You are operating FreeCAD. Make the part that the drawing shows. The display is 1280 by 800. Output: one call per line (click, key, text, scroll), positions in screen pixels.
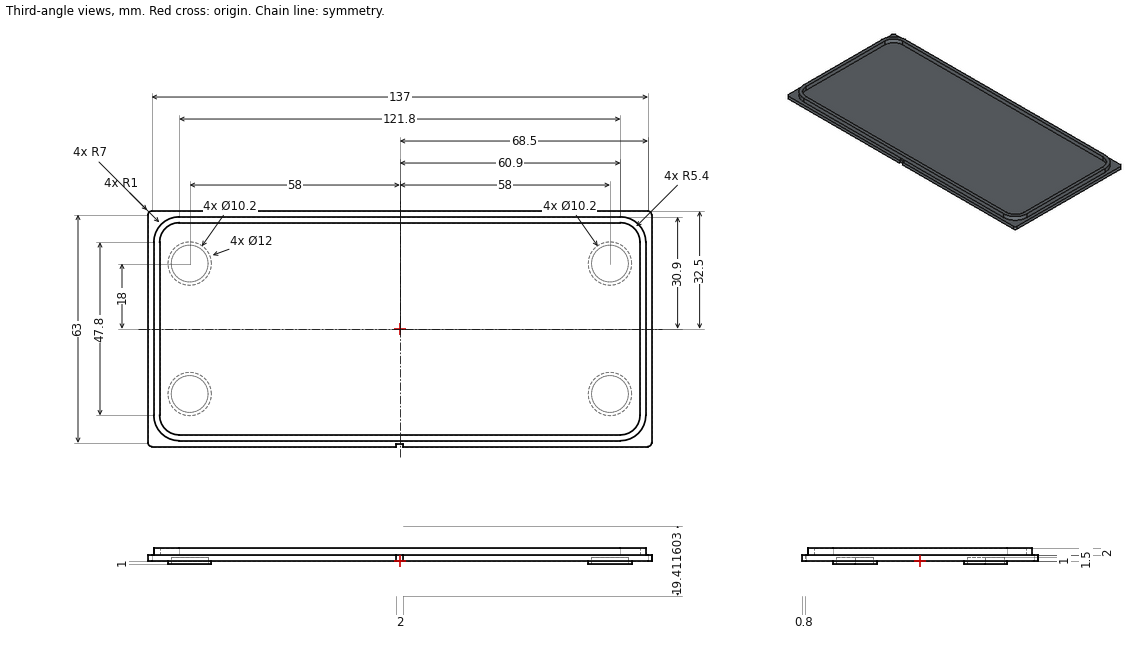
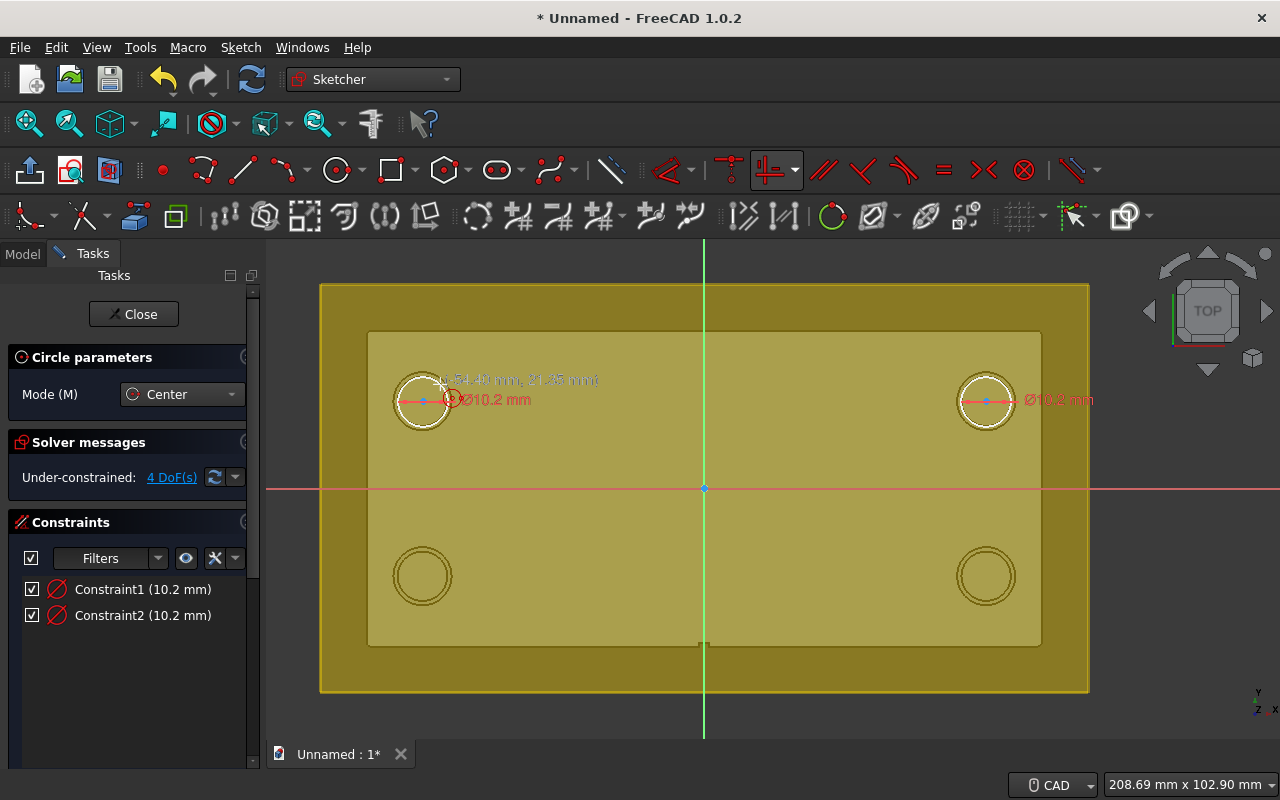
click(423, 576)
move(440, 559)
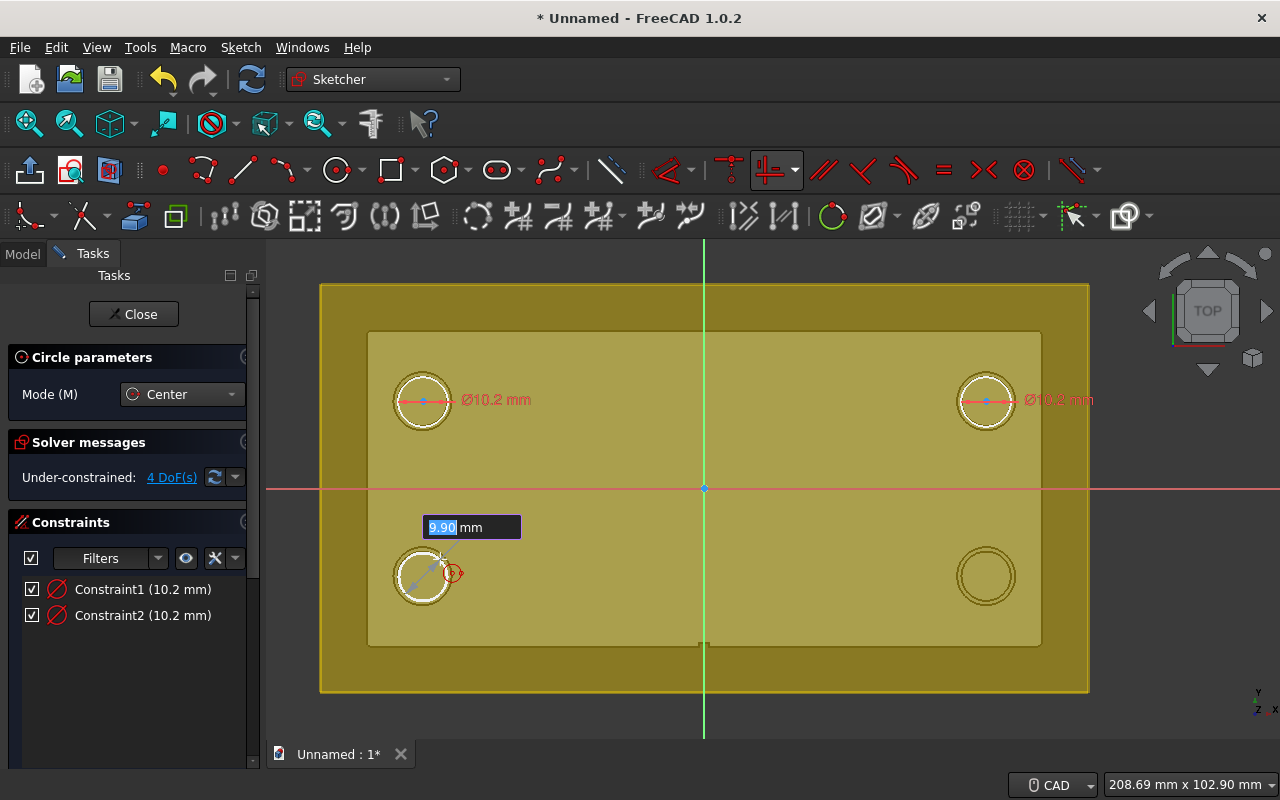
text(10.2)
key(Return)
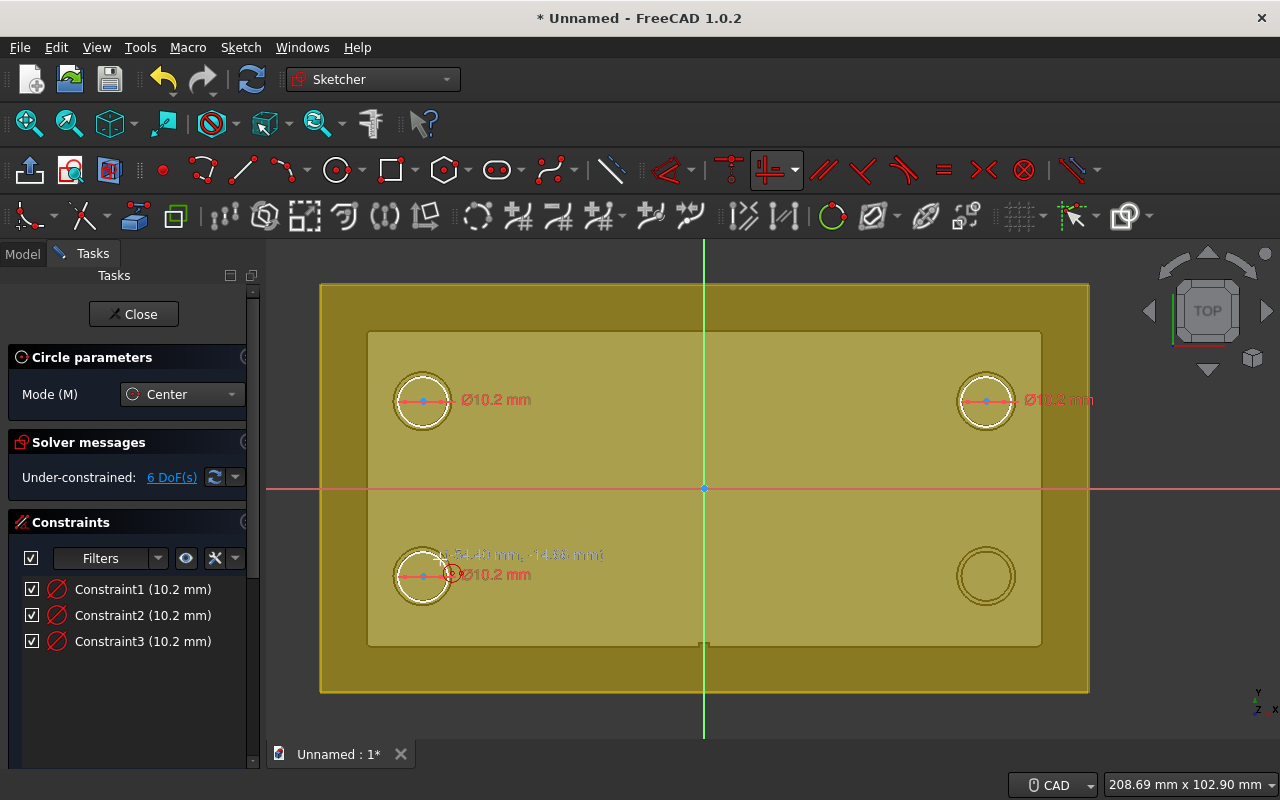
click(986, 576)
move(1004, 559)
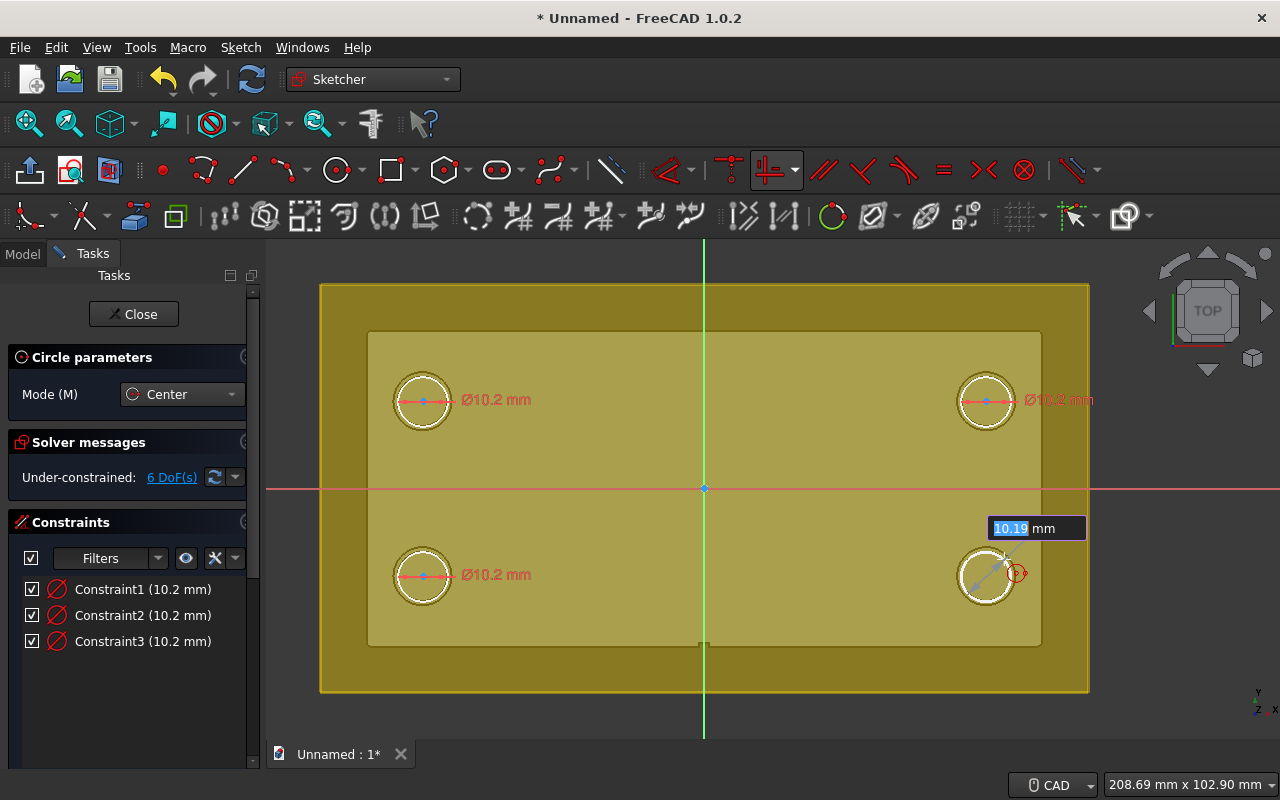
text(10.2)
key(Return)
key(Escape)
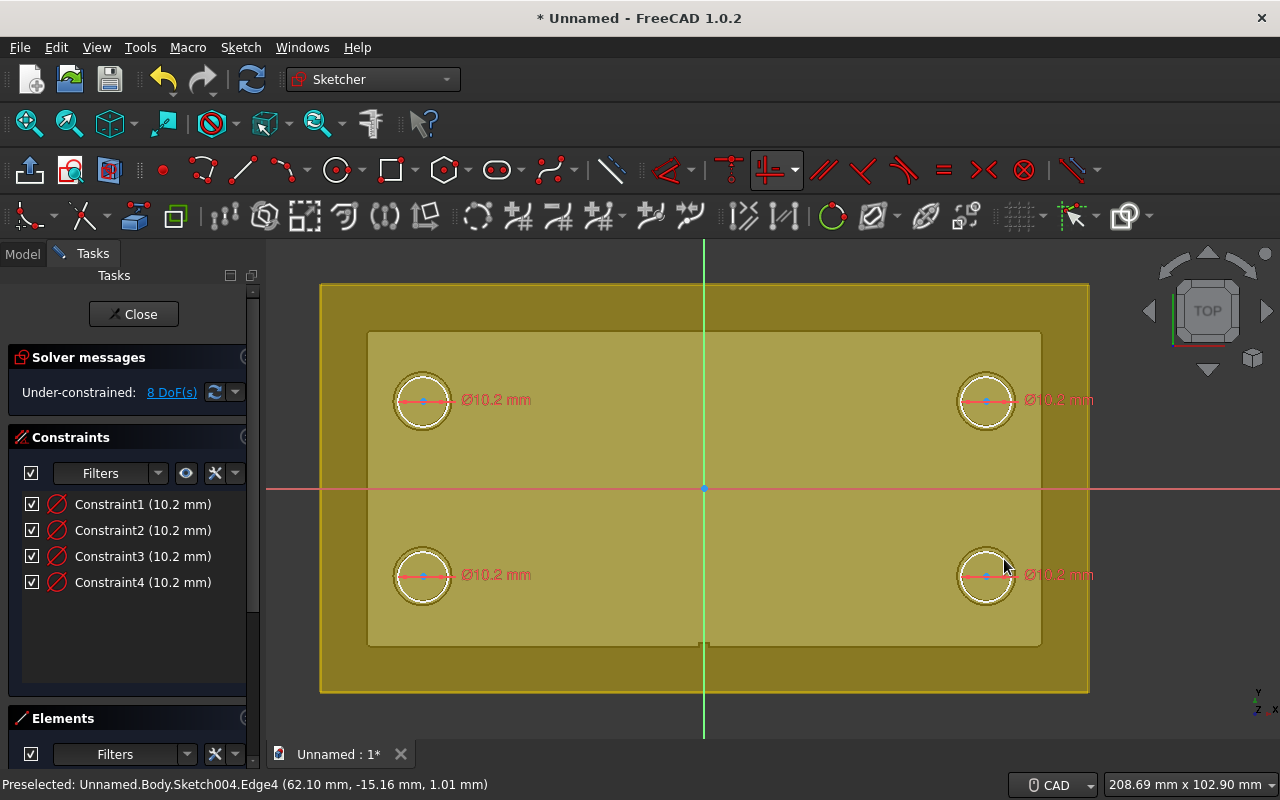
click(986, 402)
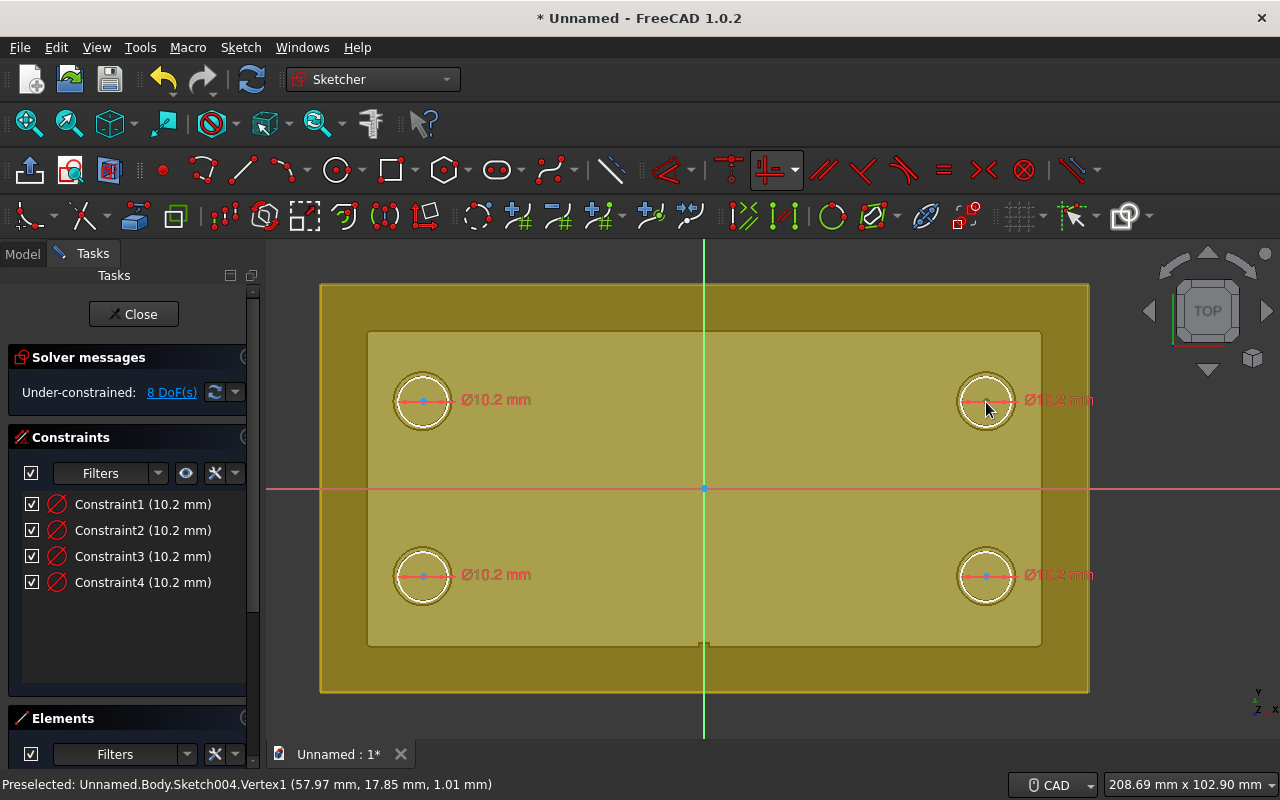
click(423, 402)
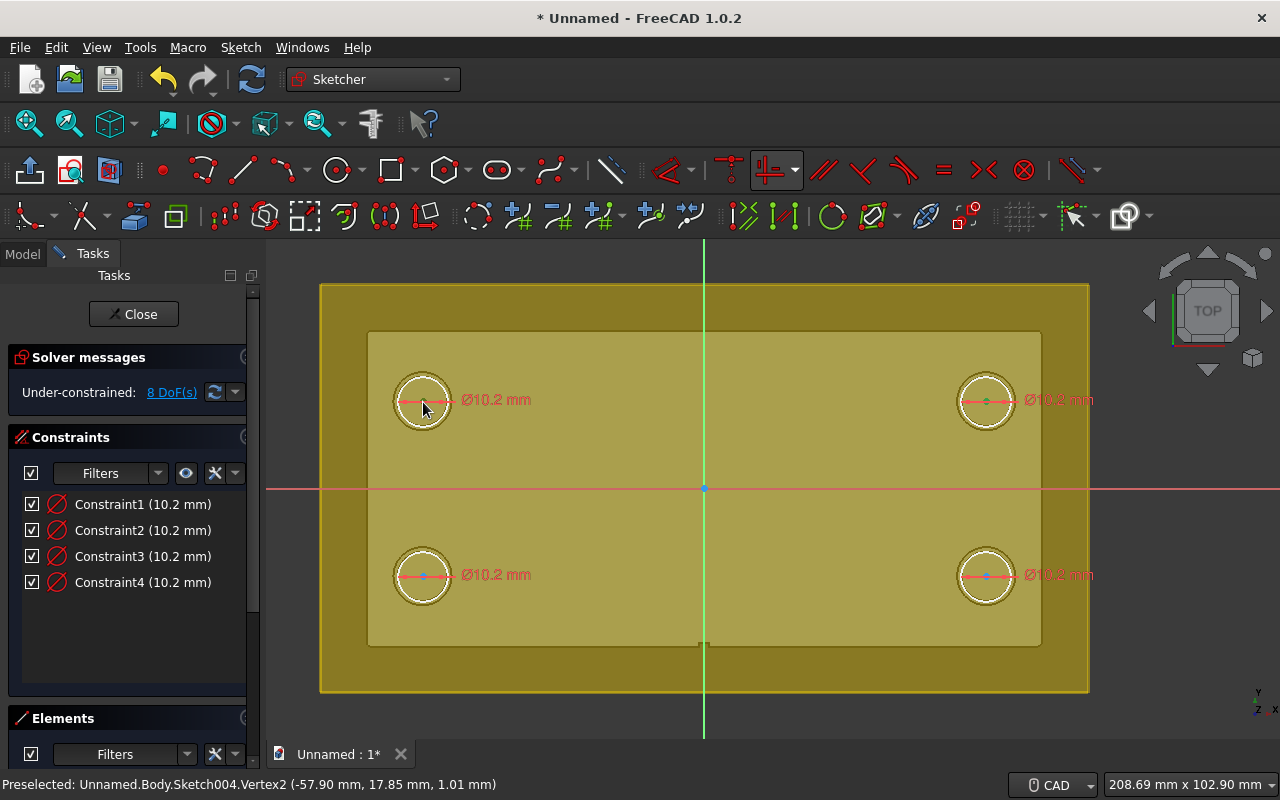
click(704, 679)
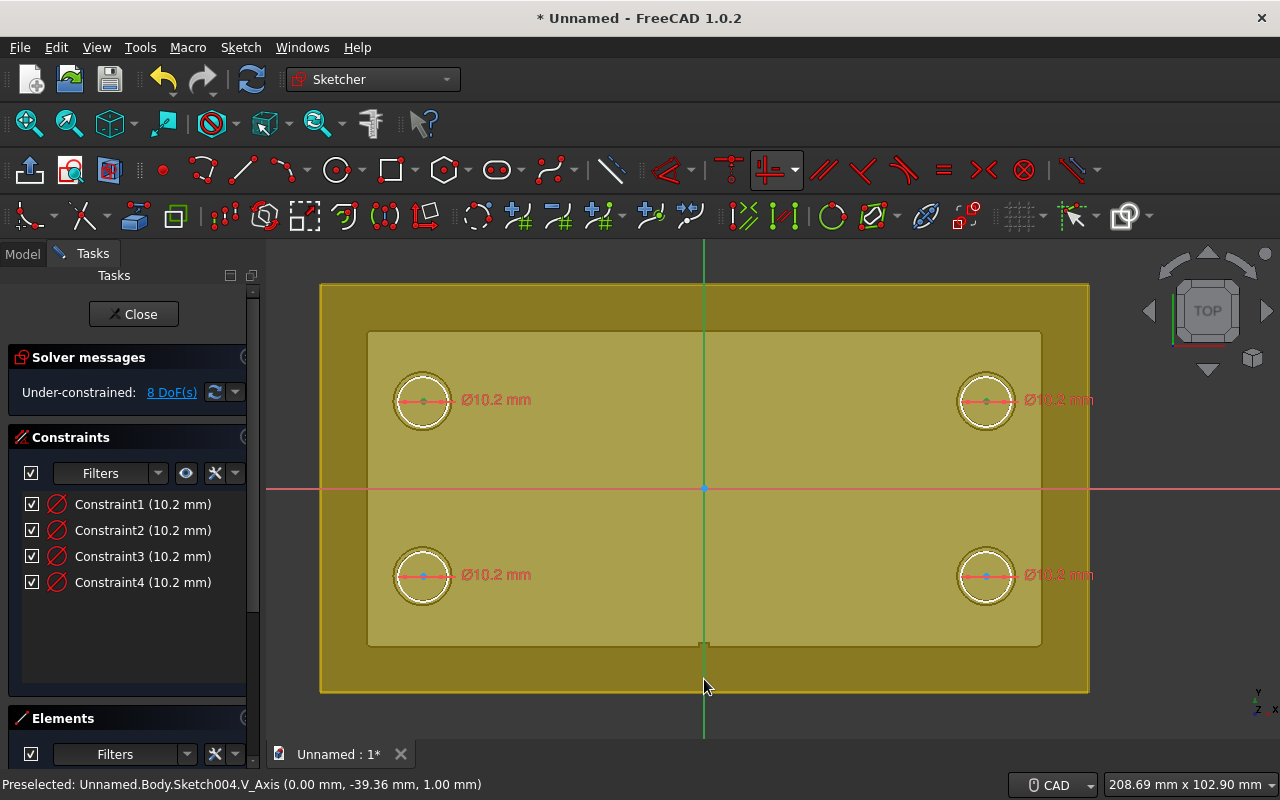
click(984, 170)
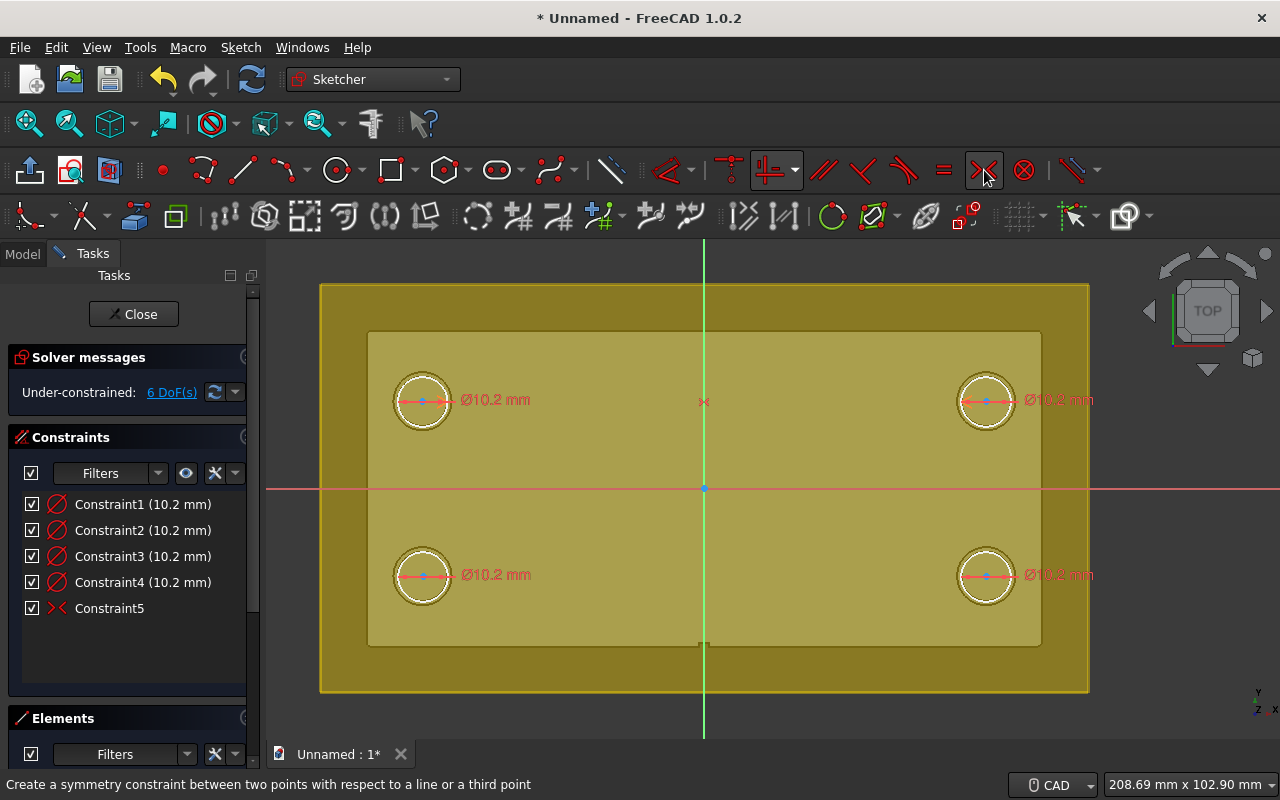
click(423, 402)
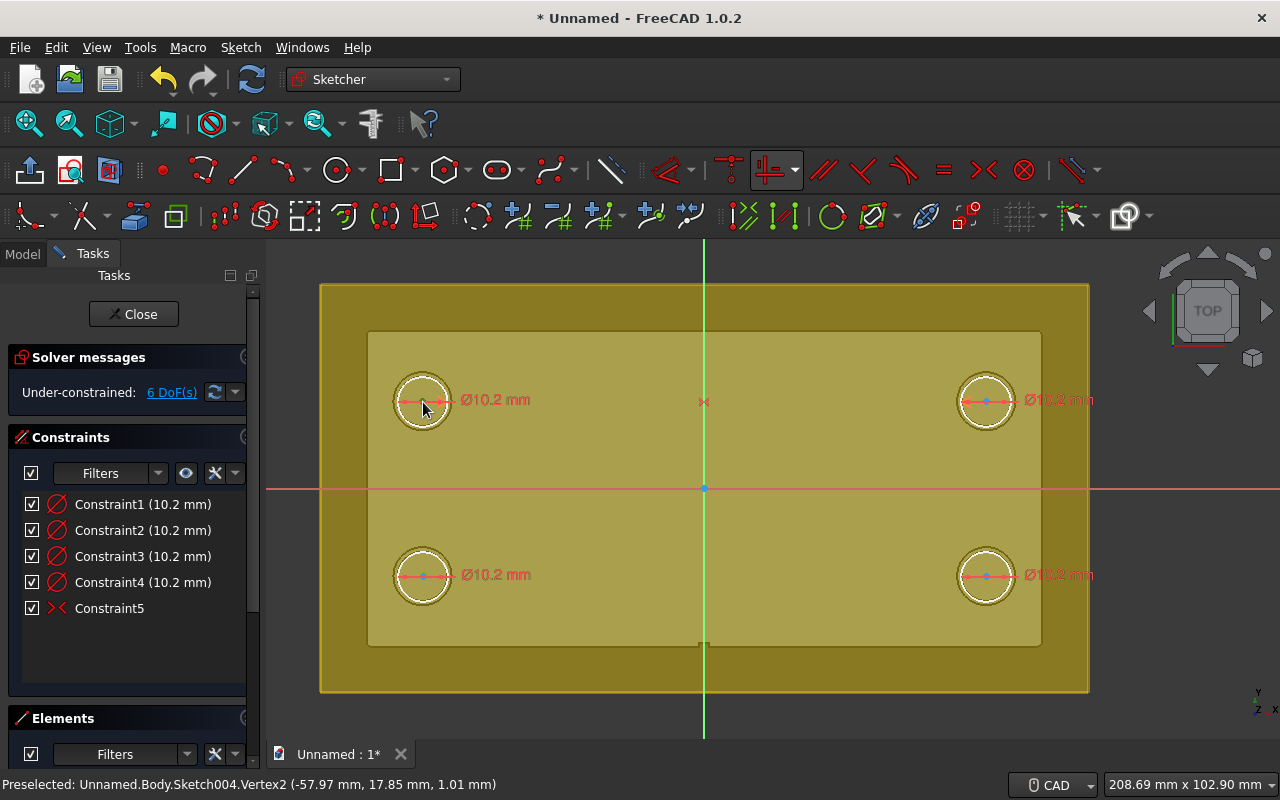
click(423, 577)